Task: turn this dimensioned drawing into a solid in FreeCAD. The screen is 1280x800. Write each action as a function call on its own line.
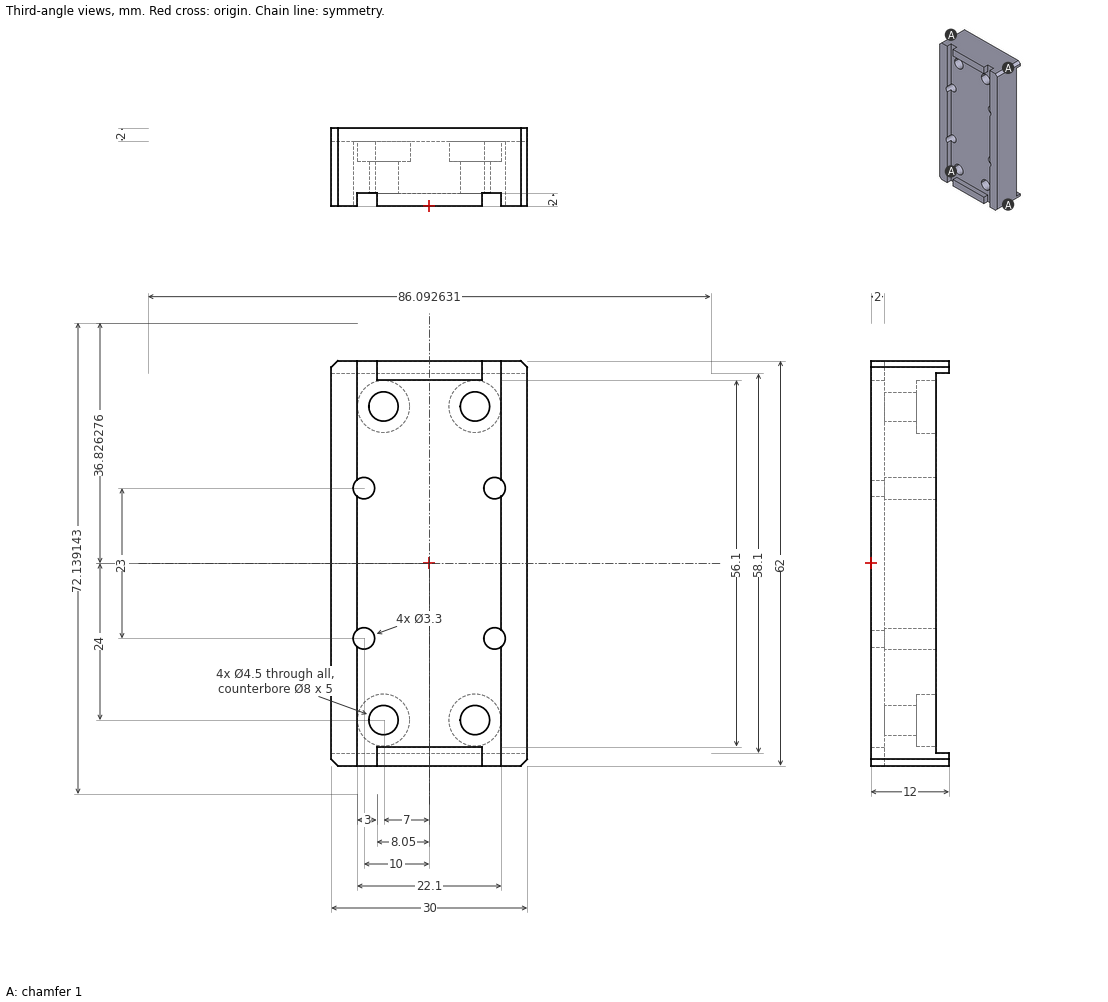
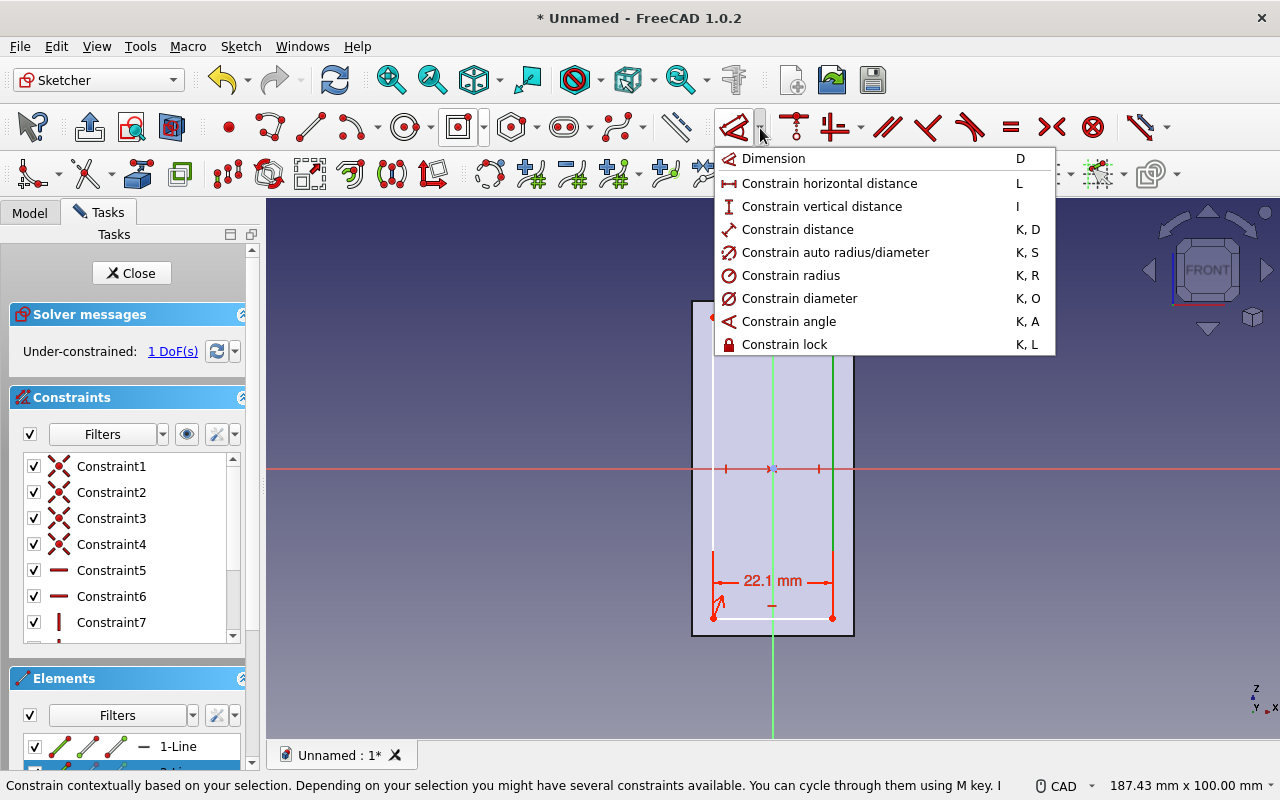
click(885, 206)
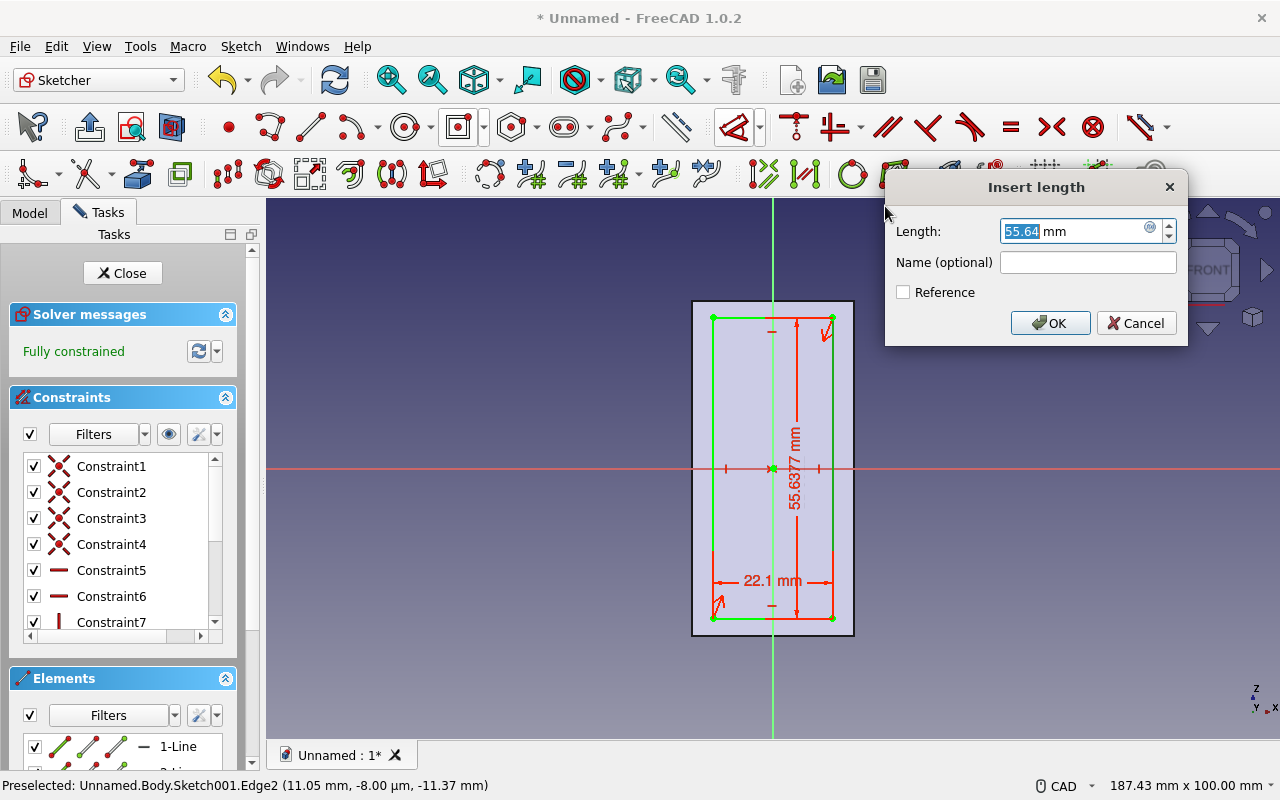
text(56.1)
key(Return)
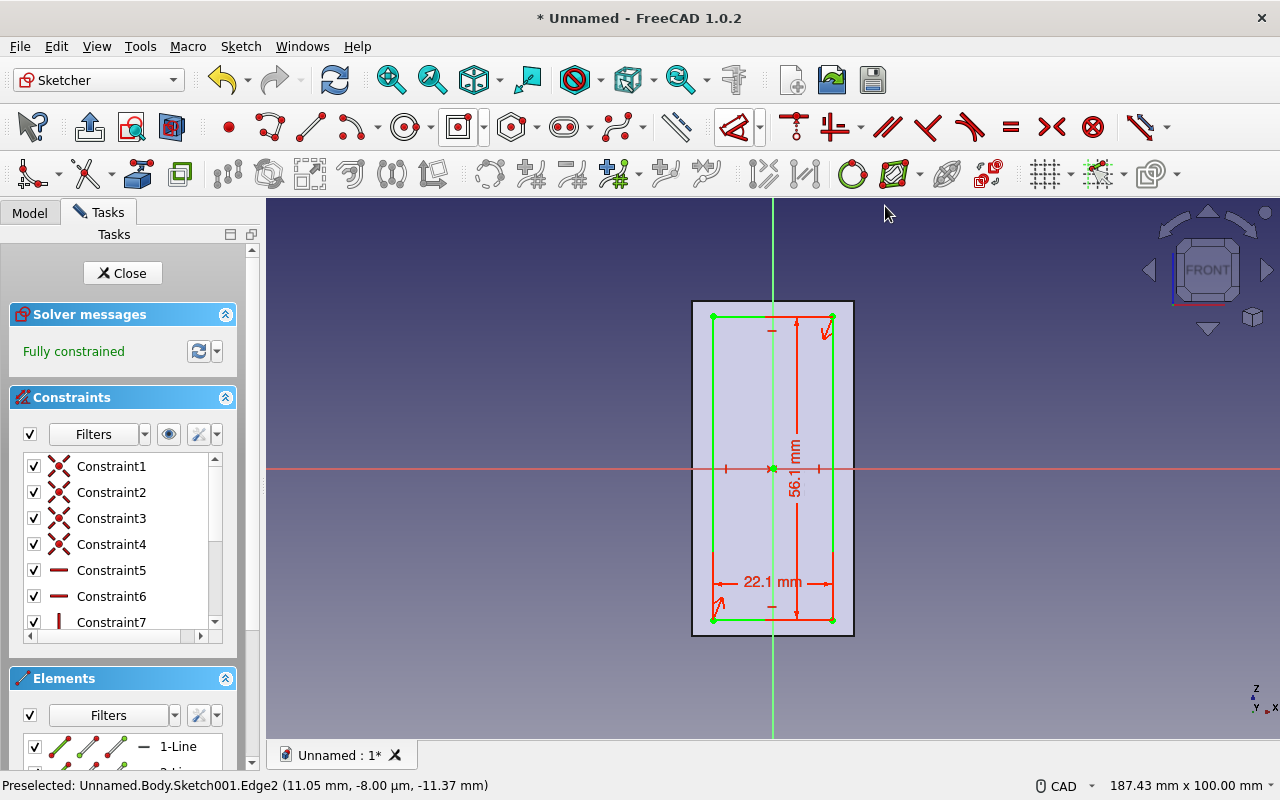
click(123, 273)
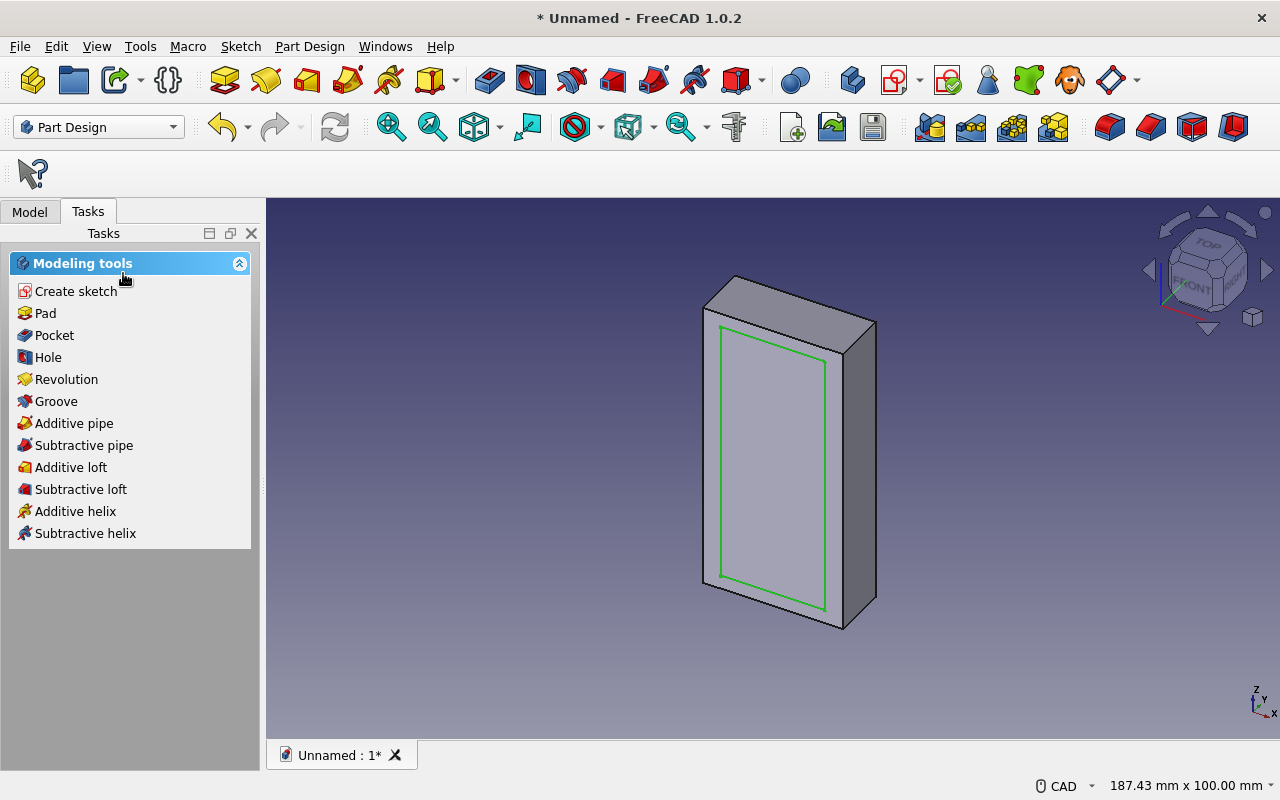
click(490, 80)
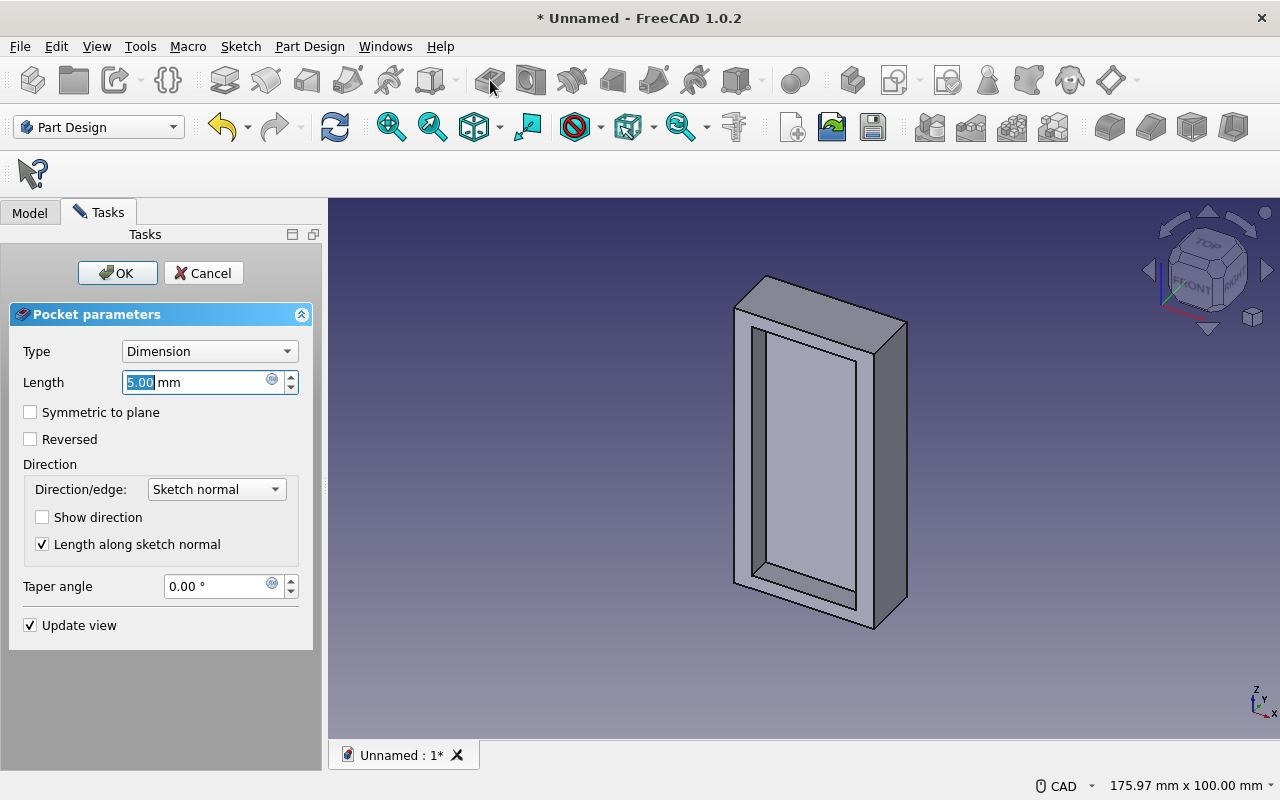
text(2)
key(Tab)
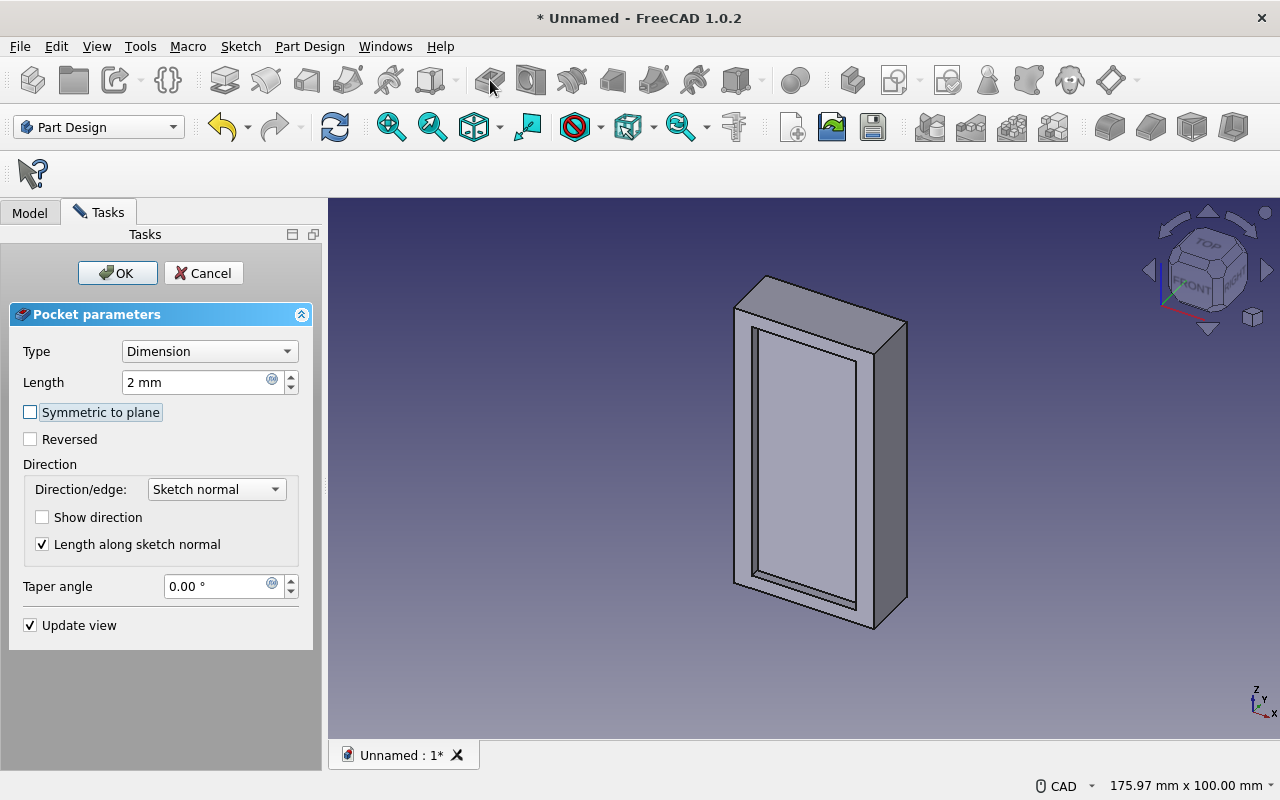
click(118, 273)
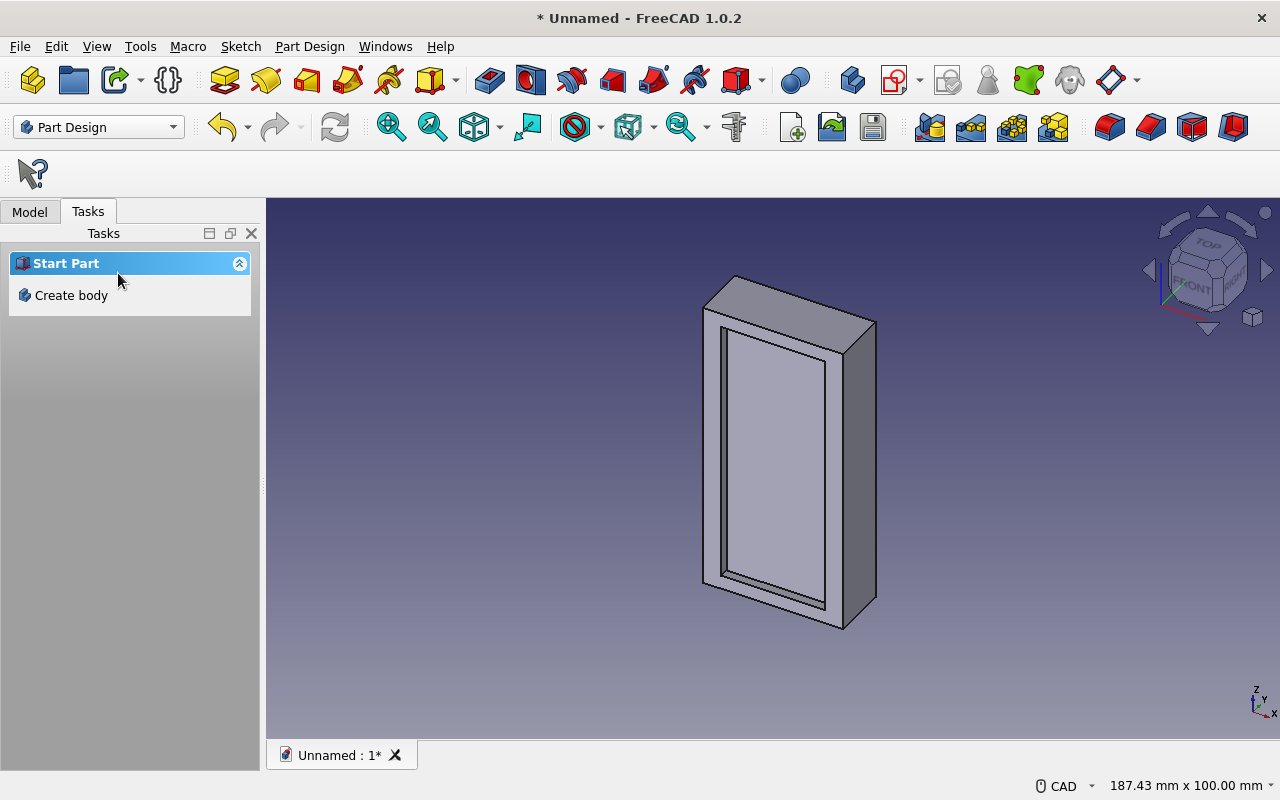
click(894, 80)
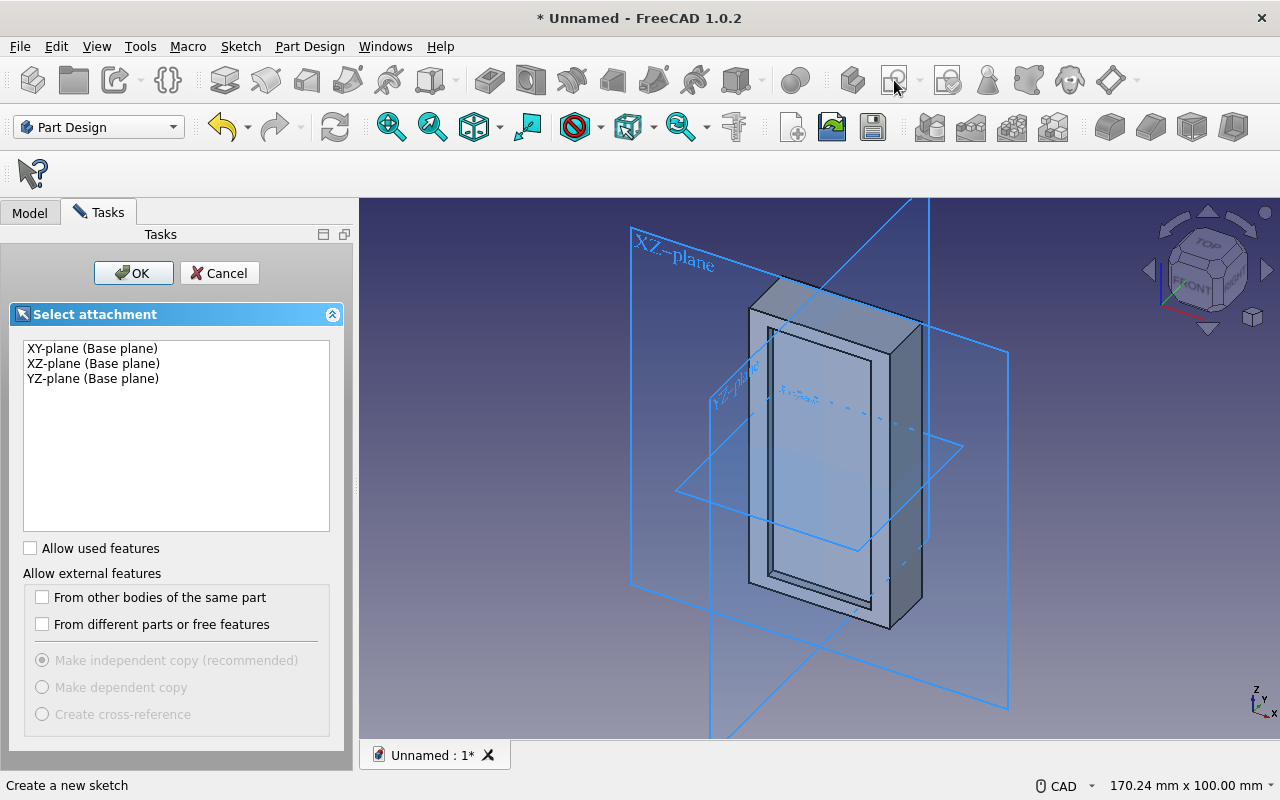
click(84, 364)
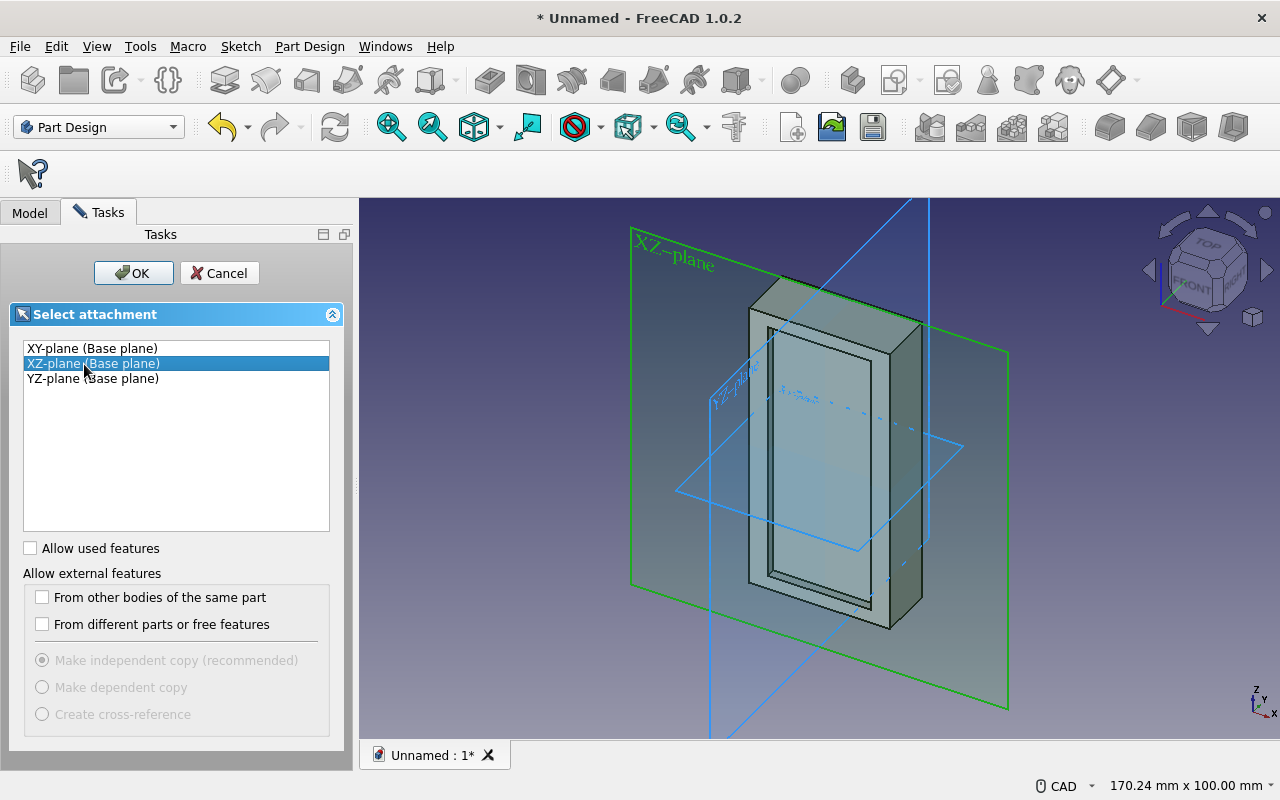
click(134, 273)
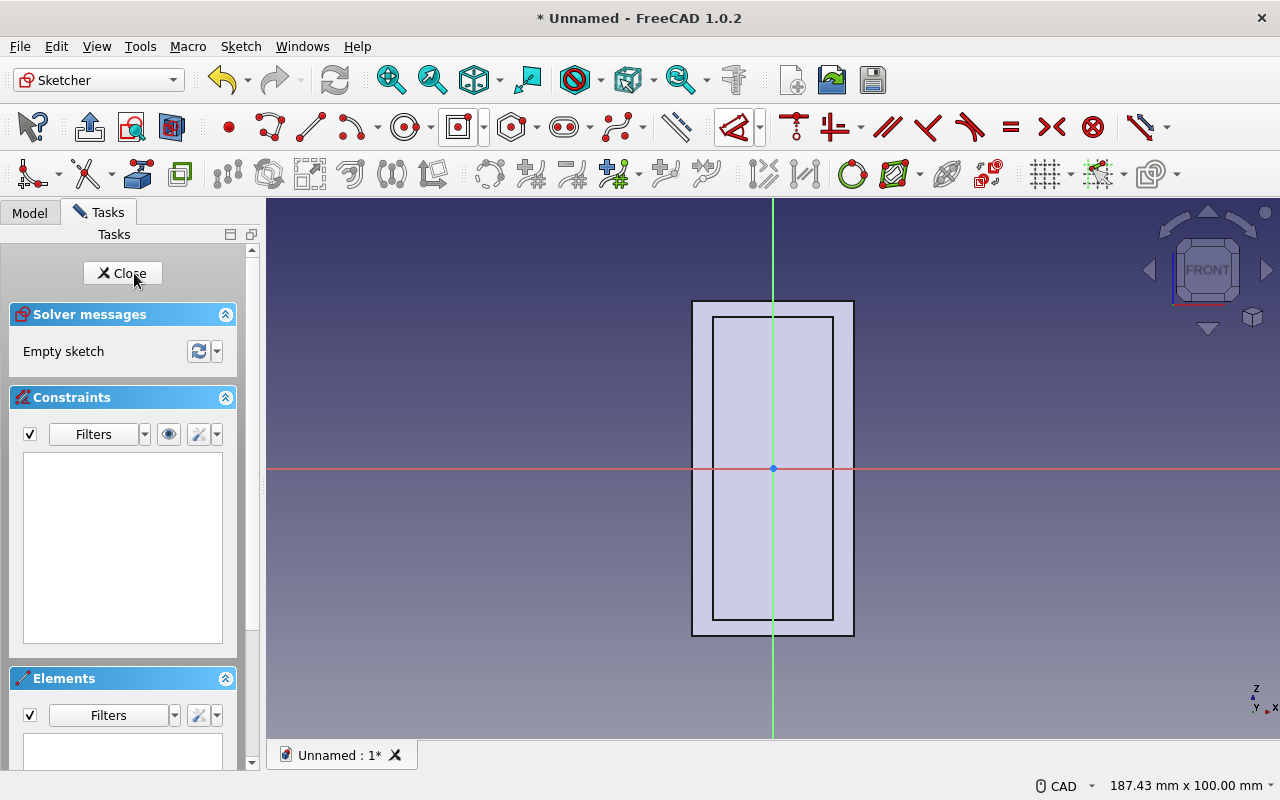
click(484, 128)